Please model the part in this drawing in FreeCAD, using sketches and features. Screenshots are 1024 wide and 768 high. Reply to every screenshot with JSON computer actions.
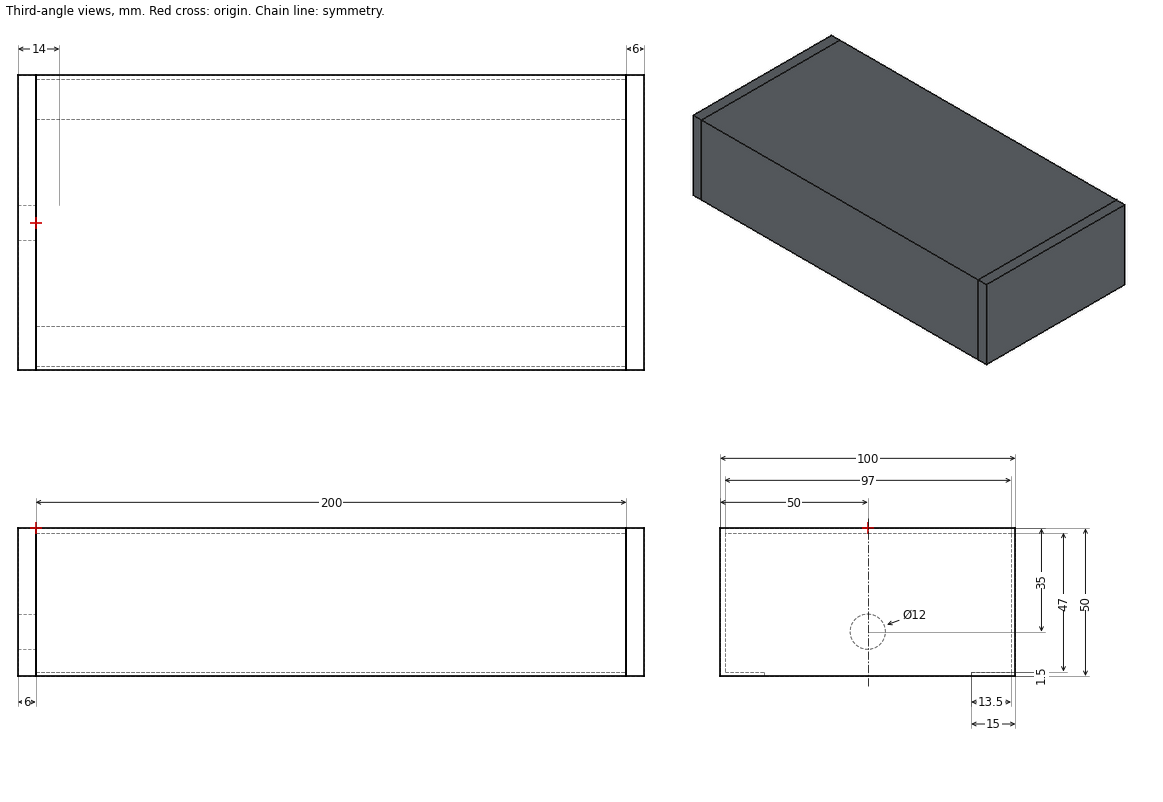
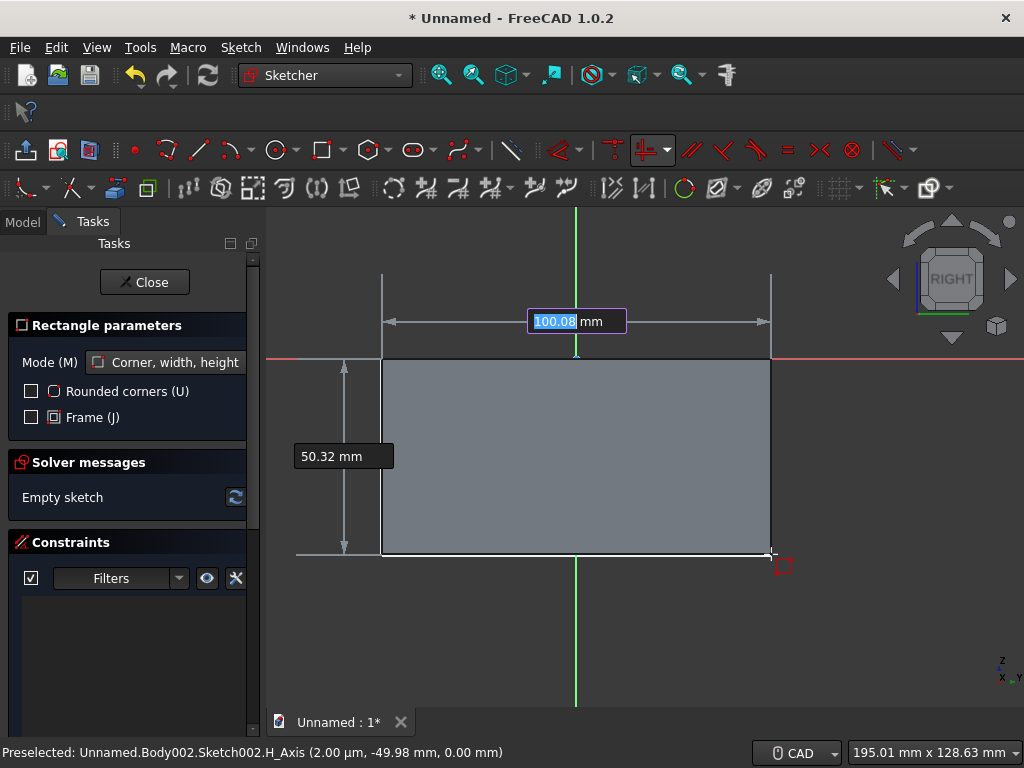
{"action": "type", "text": "100"}
{"action": "key", "text": "Tab"}
{"action": "type", "text": "50"}
{"action": "key", "text": "Return"}
{"action": "key", "text": "Escape"}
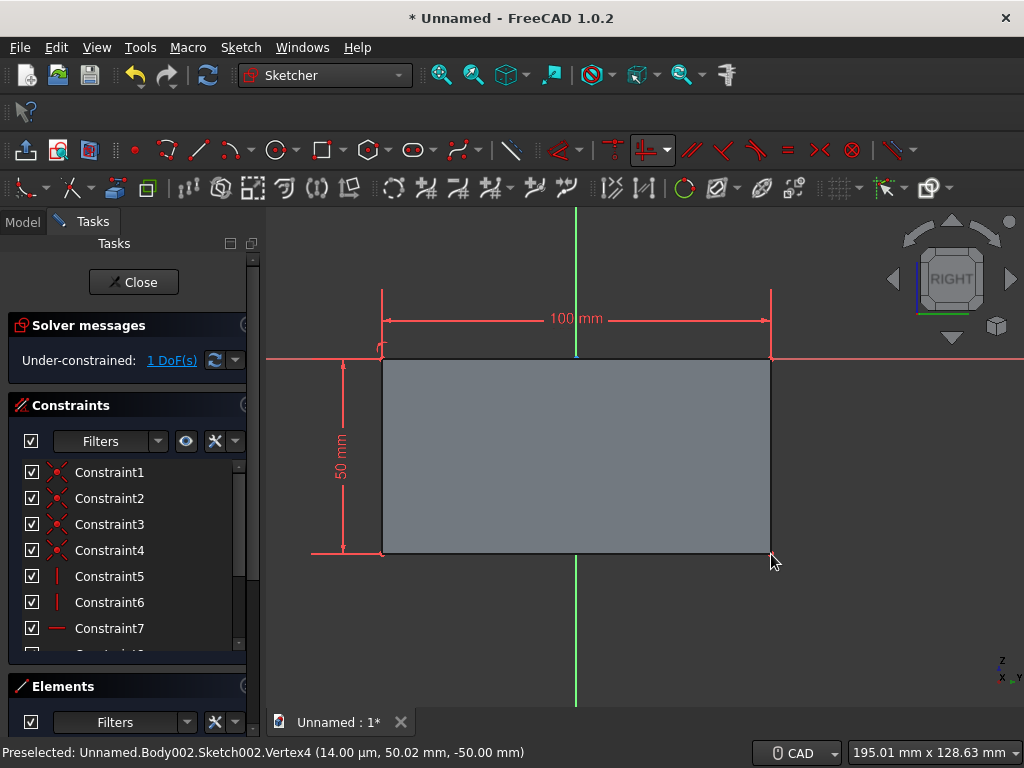
{"action": "left_click", "coordinate": [558, 150]}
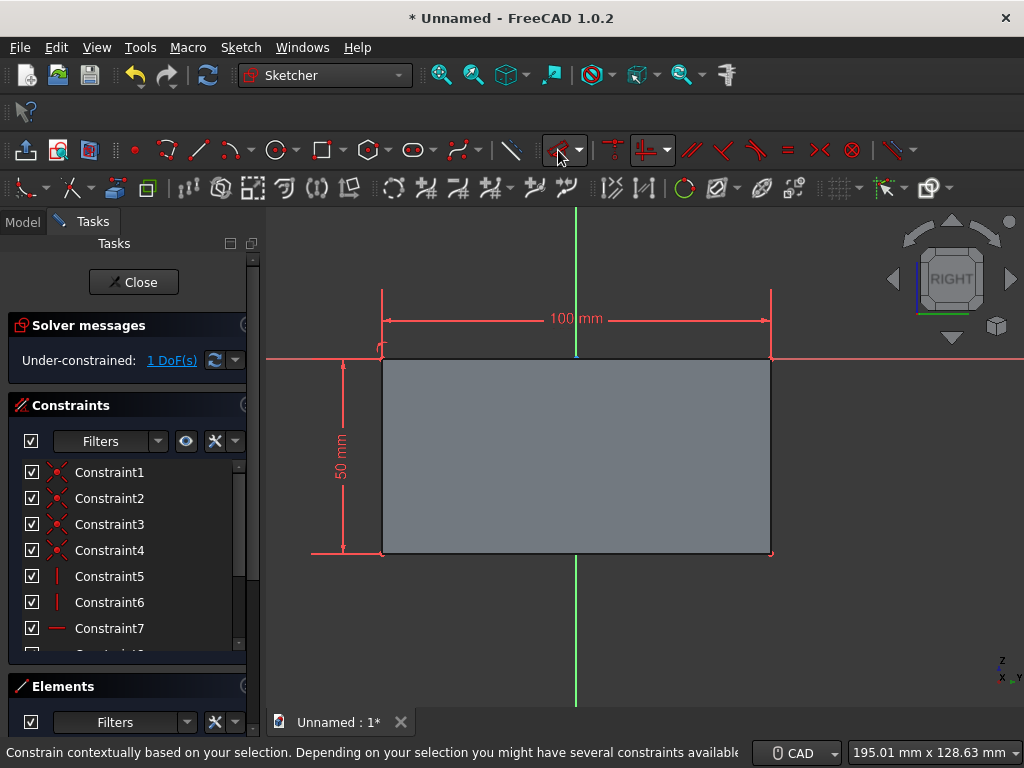
{"action": "left_click", "coordinate": [382, 359]}
{"action": "left_click", "coordinate": [479, 325]}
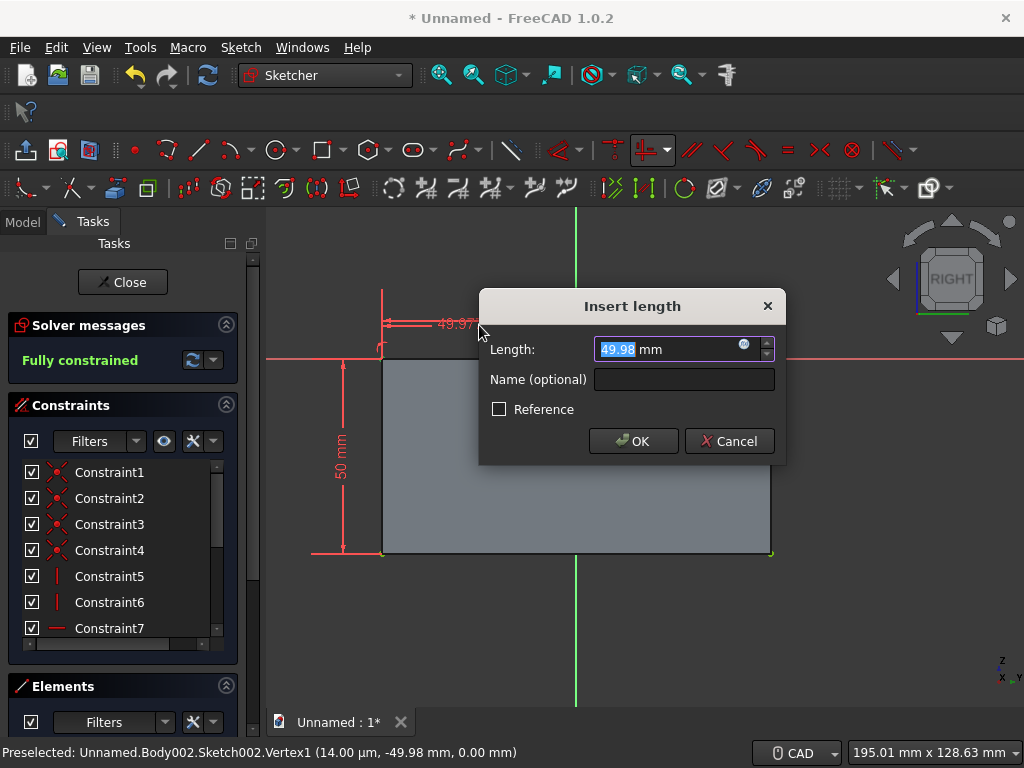
{"action": "type", "text": "50"}
{"action": "key", "text": "Return"}
{"action": "key", "text": "Escape"}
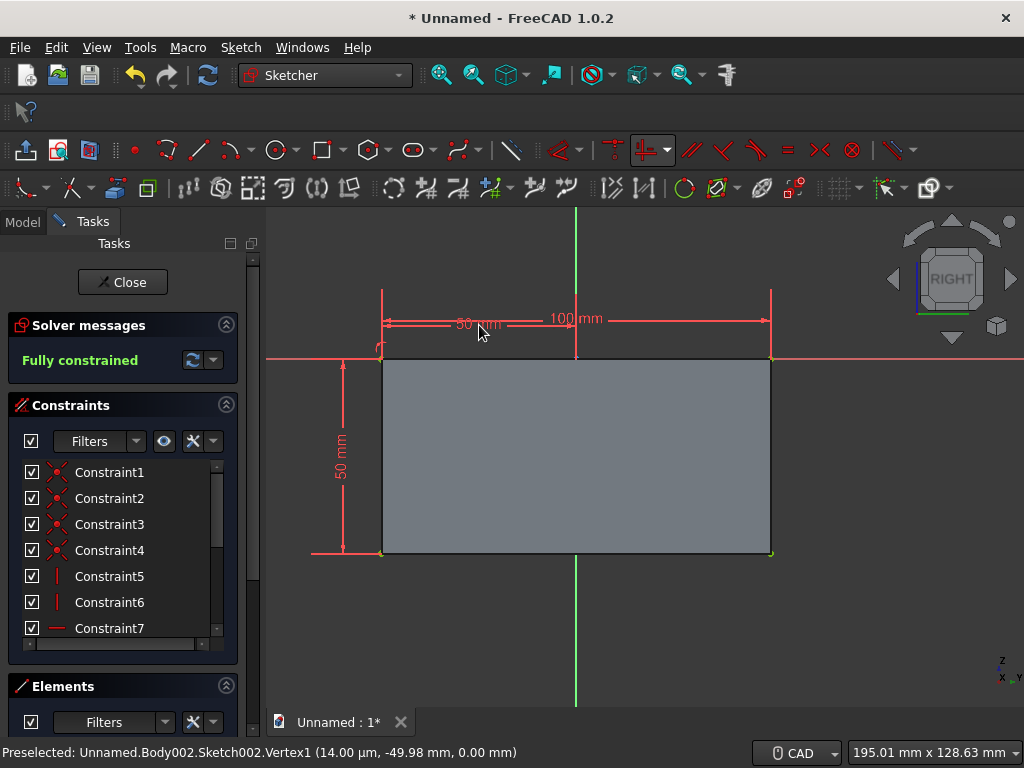
{"action": "left_click", "coordinate": [123, 282]}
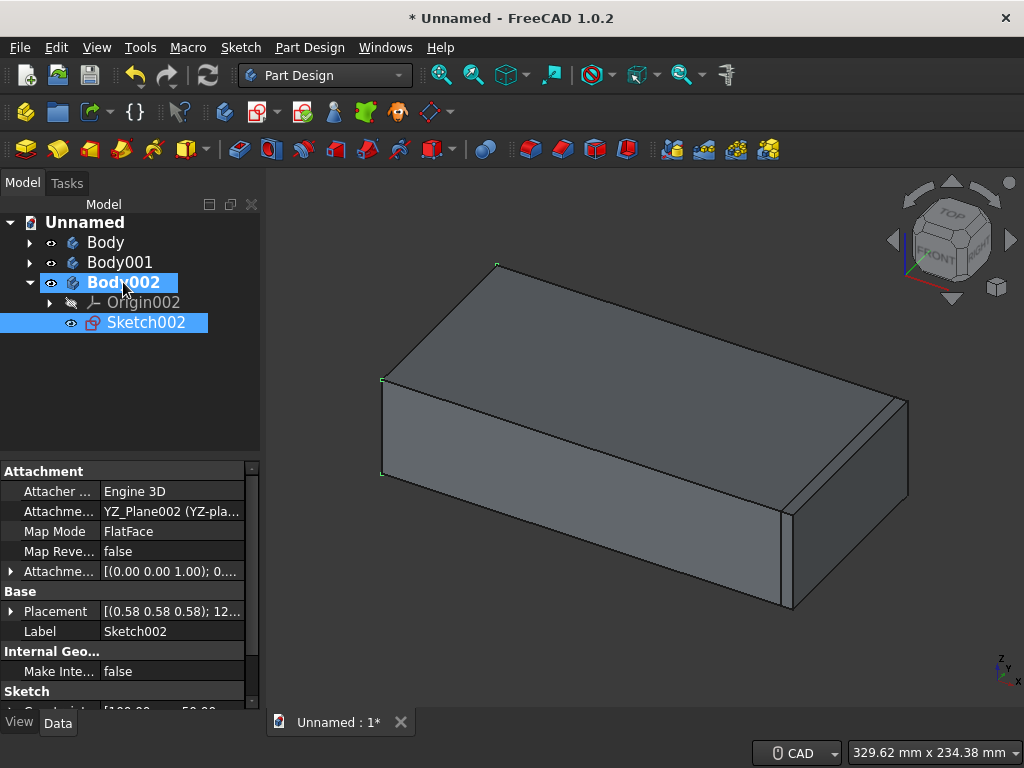
{"action": "left_click", "coordinate": [26, 150]}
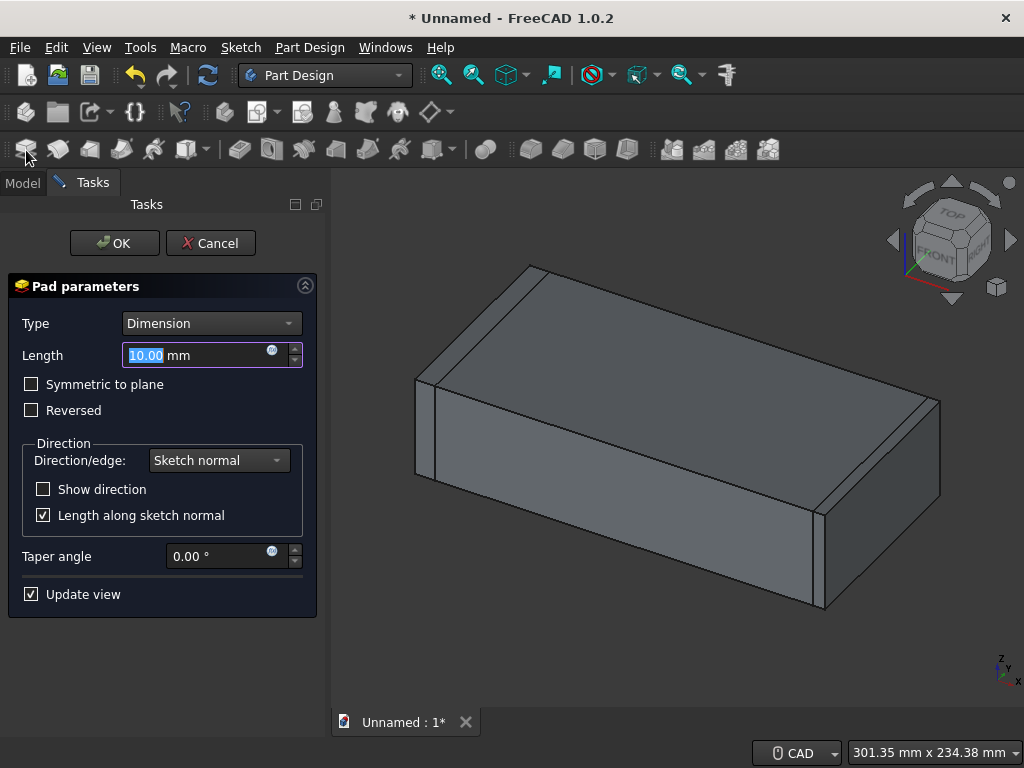
{"action": "type", "text": "6"}
{"action": "key", "text": "Tab"}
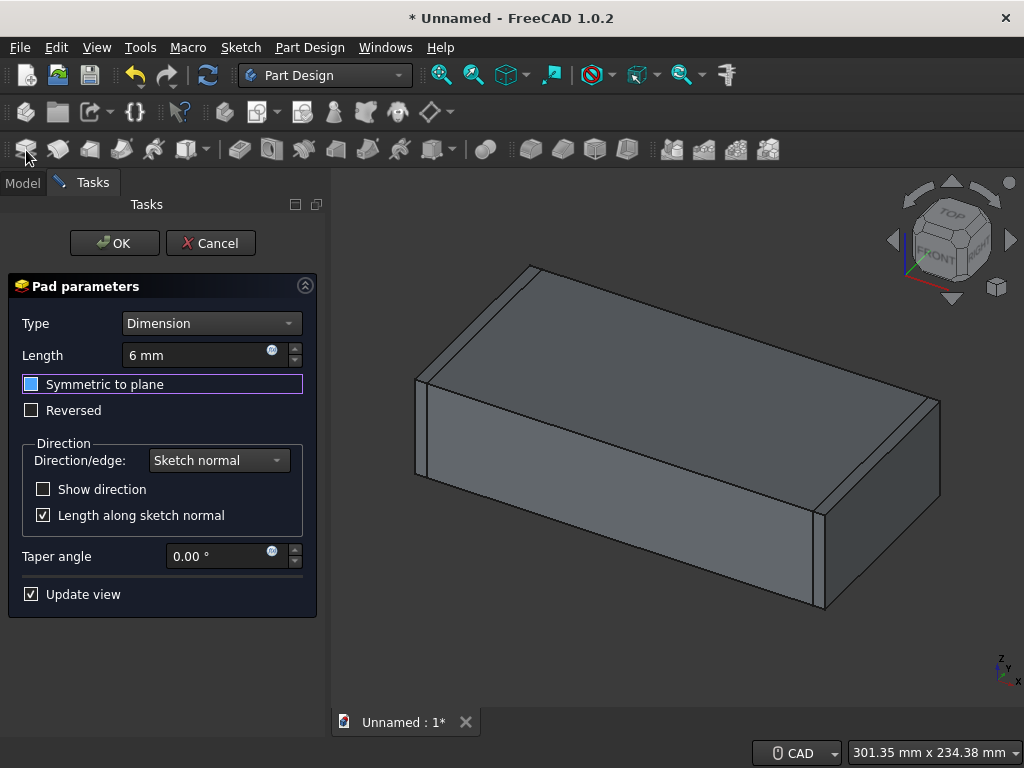
{"action": "left_click", "coordinate": [30, 410]}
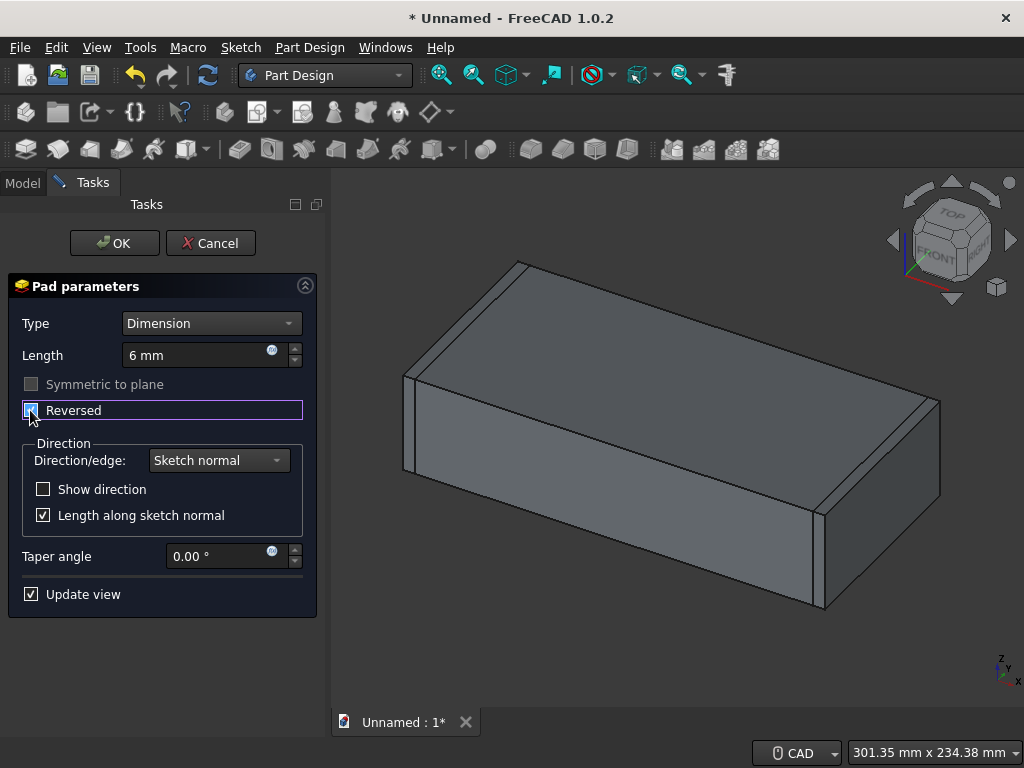
{"action": "left_click", "coordinate": [115, 243]}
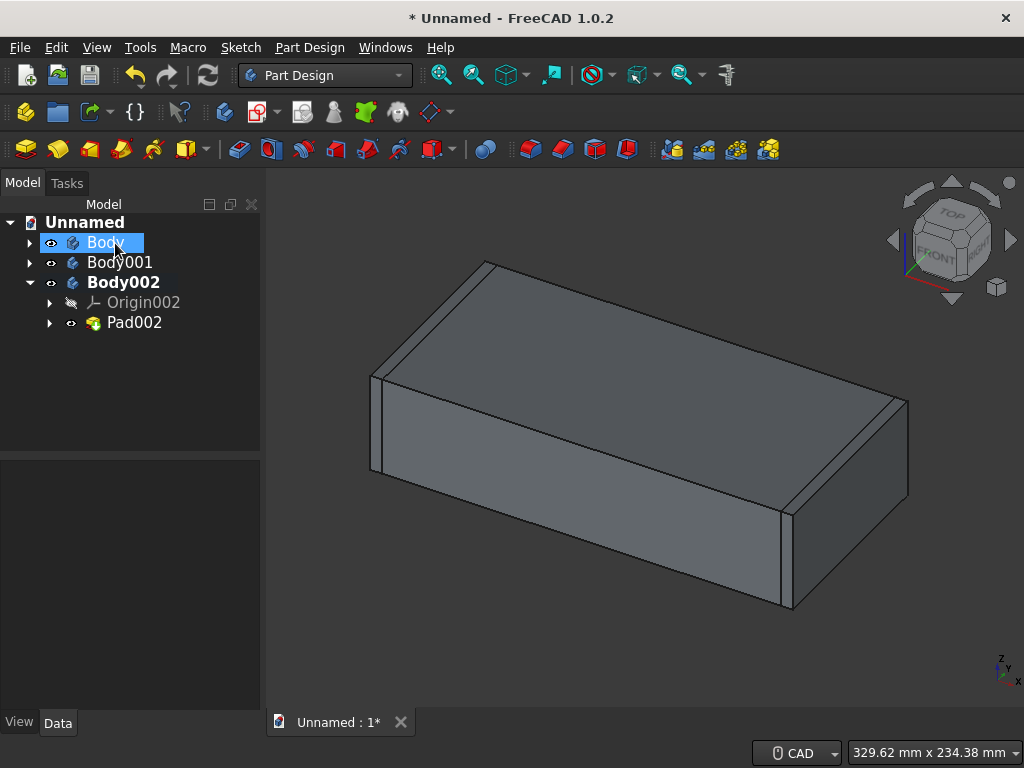
{"action": "left_click", "coordinate": [442, 76]}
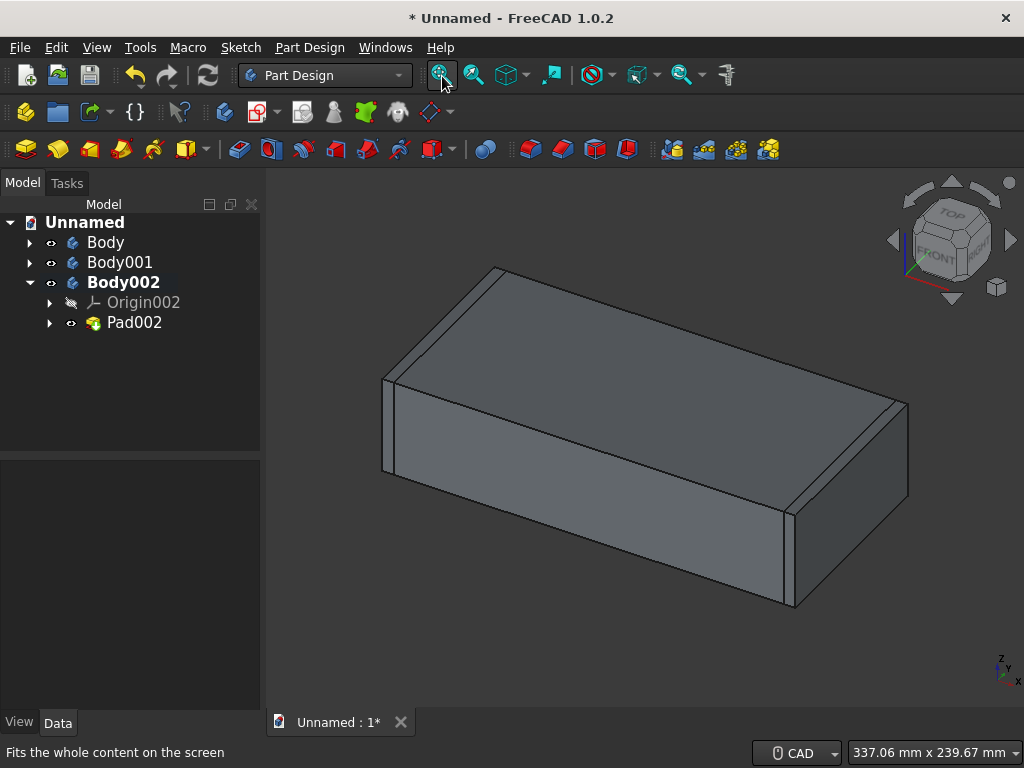
{"action": "key", "text": "6"}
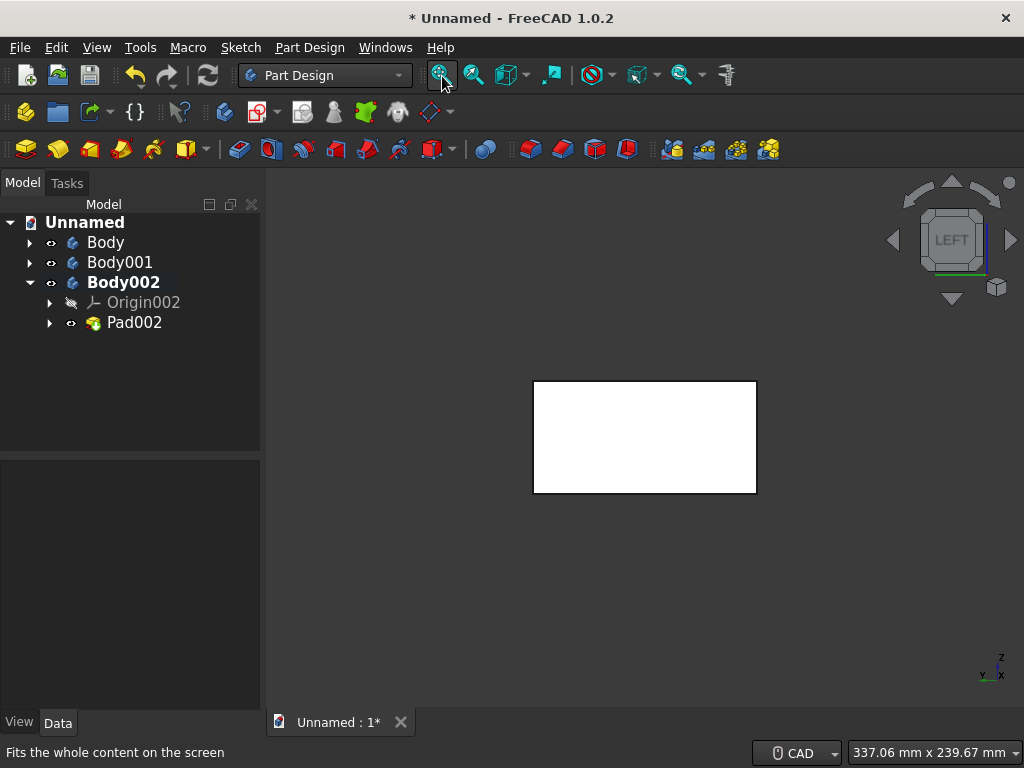
{"action": "key", "text": "v f"}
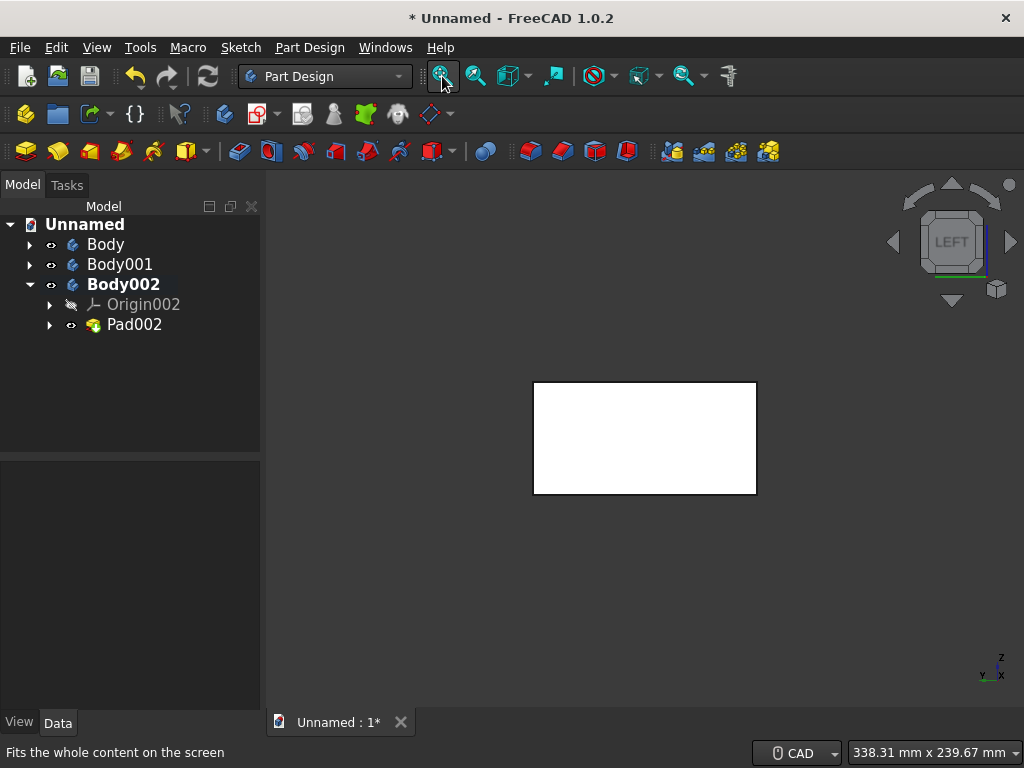
{"action": "left_click", "coordinate": [645, 437]}